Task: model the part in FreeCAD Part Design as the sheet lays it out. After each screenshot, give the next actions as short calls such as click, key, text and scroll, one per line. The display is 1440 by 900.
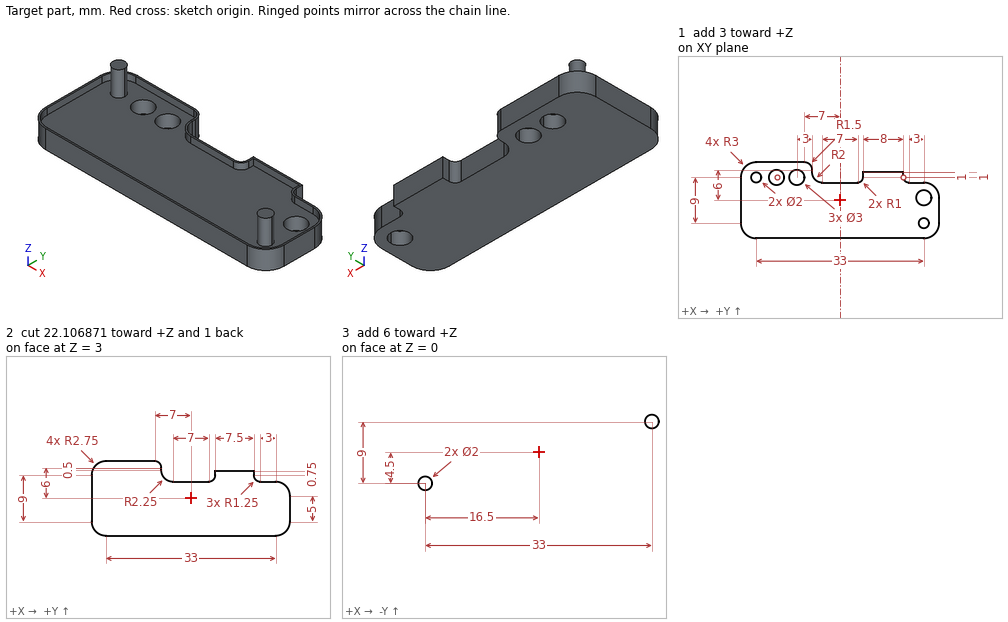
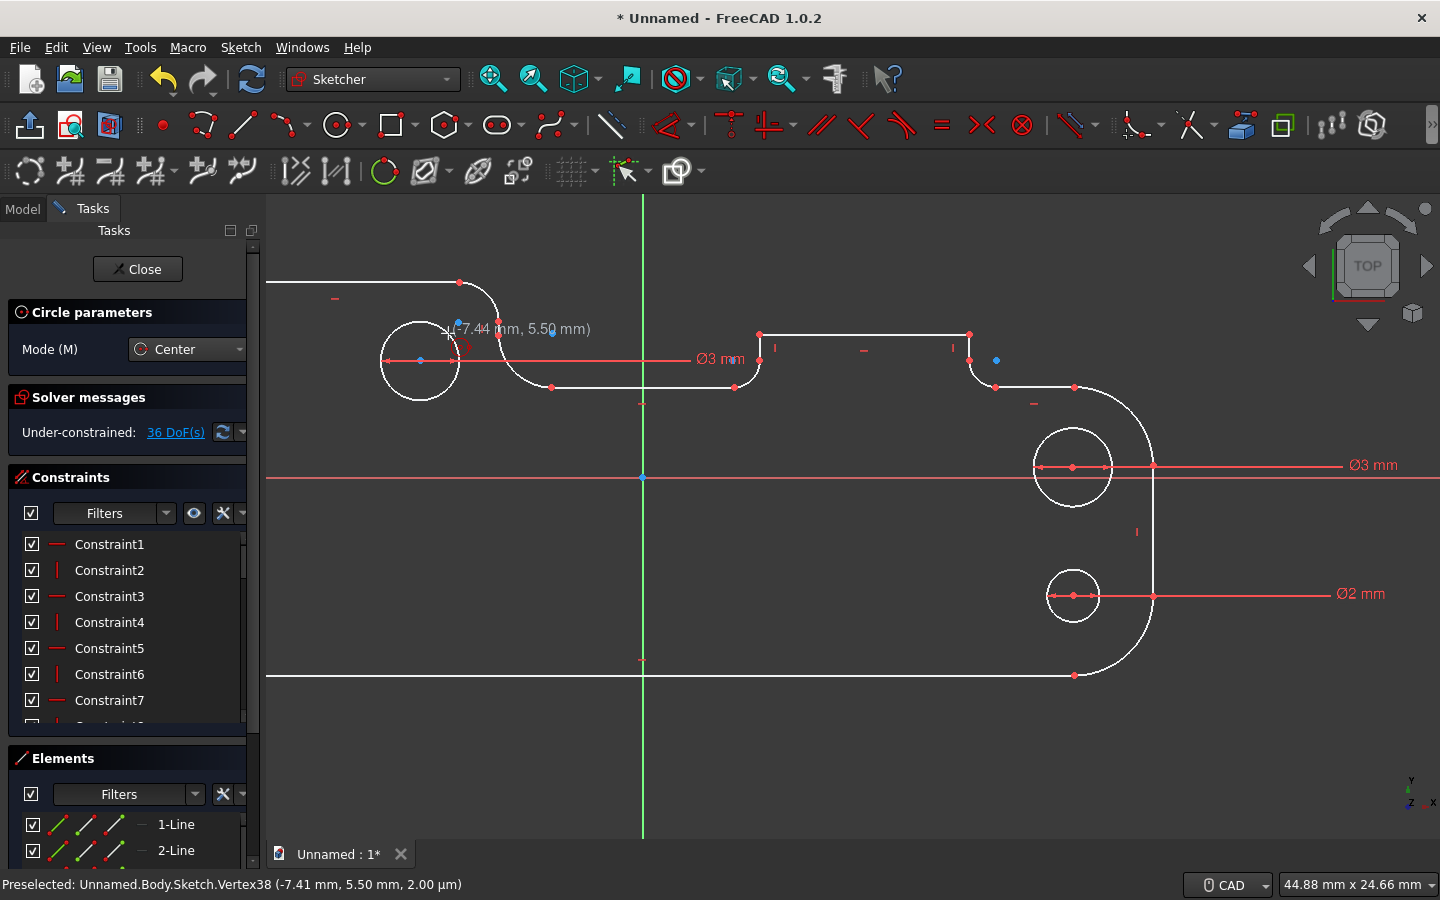
click(316, 360)
move(343, 333)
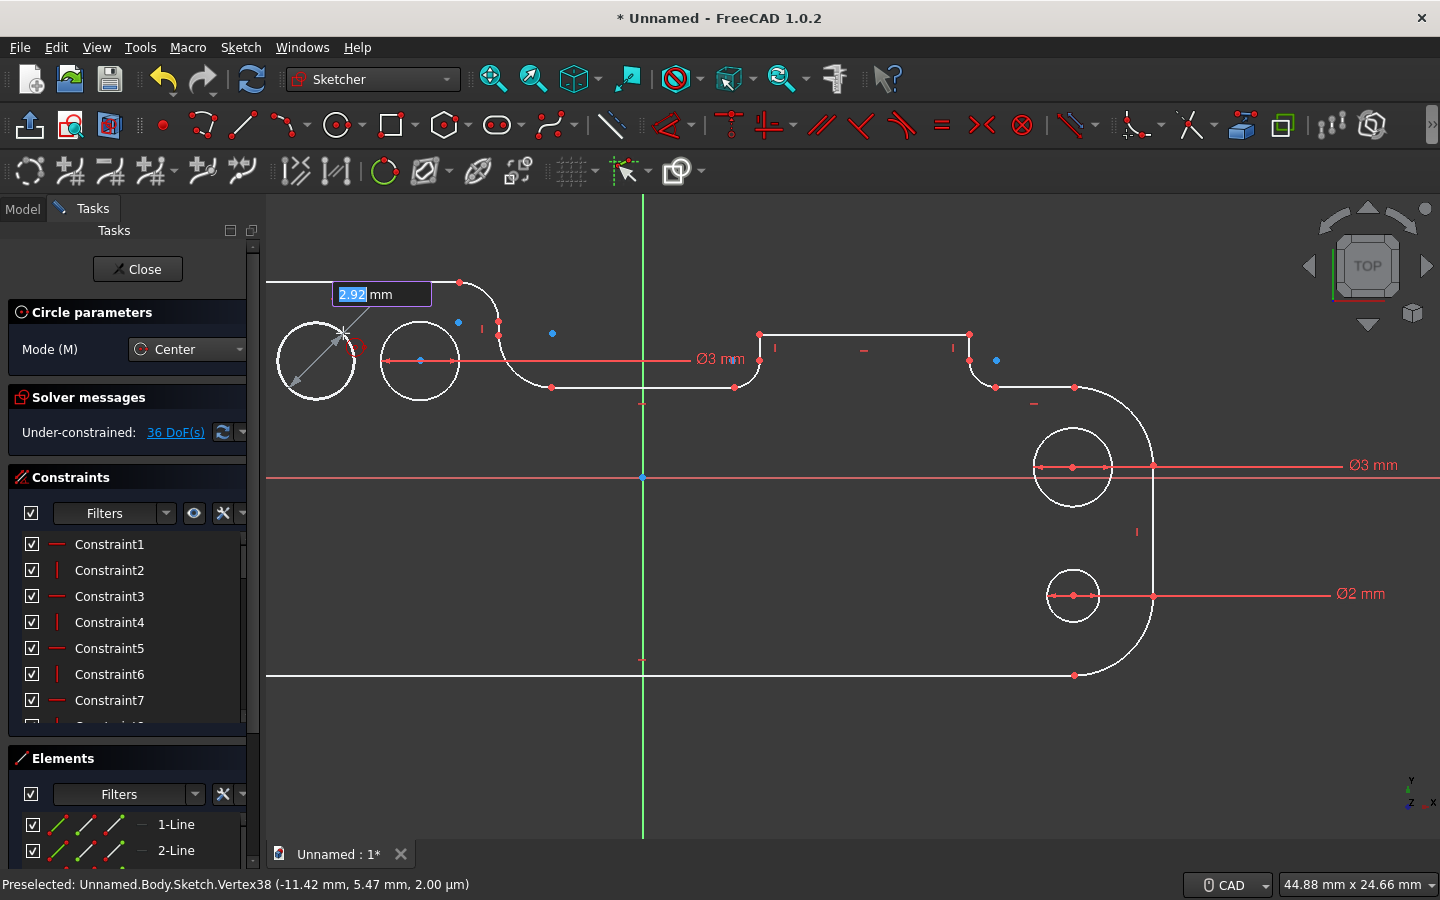
text(3)
key(Return)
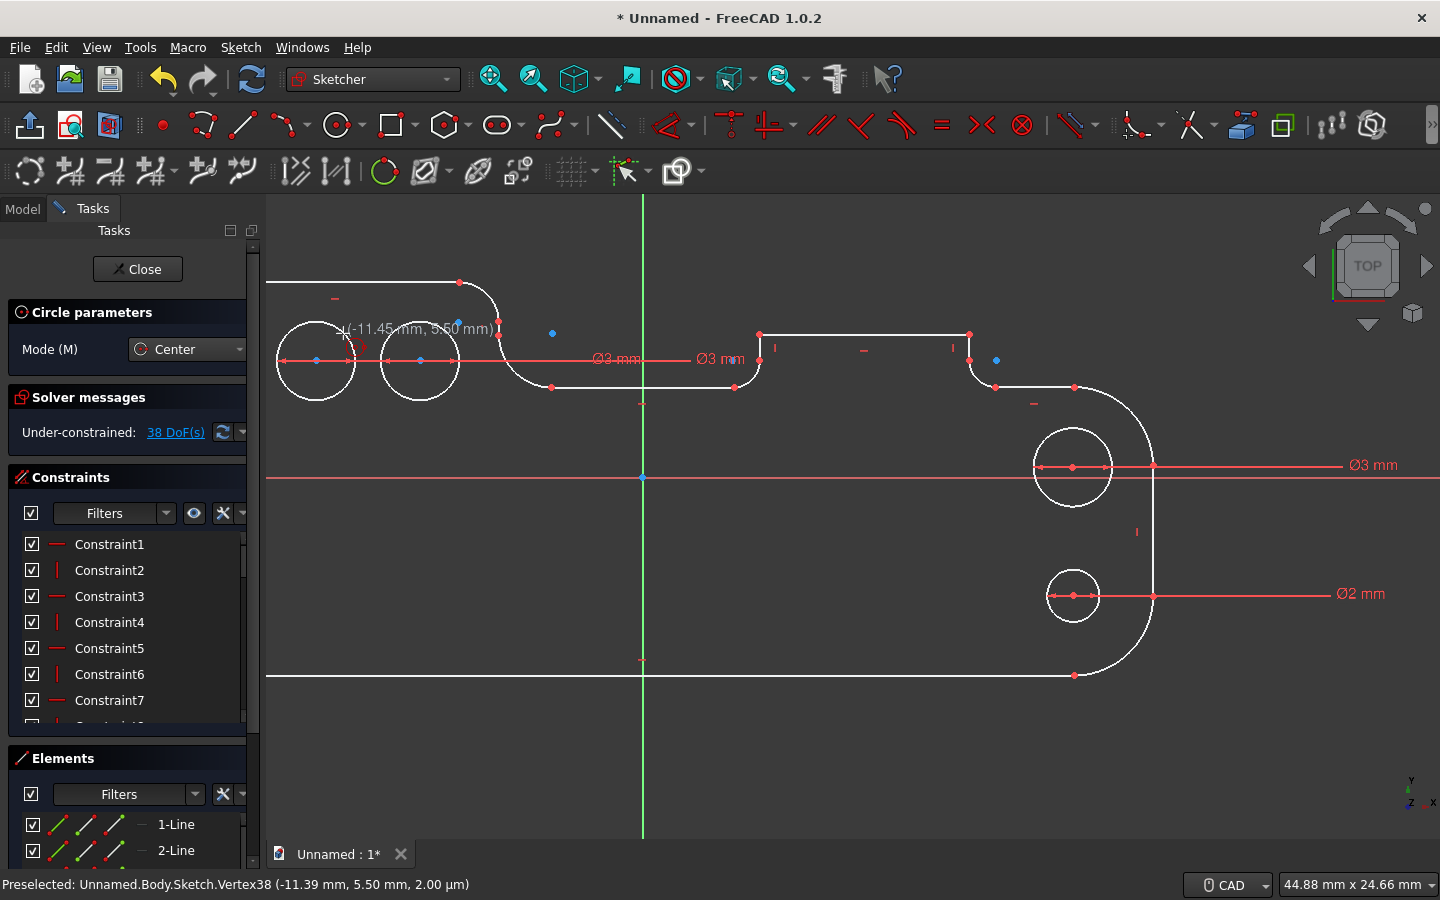
scroll(1073, 595, down, 2)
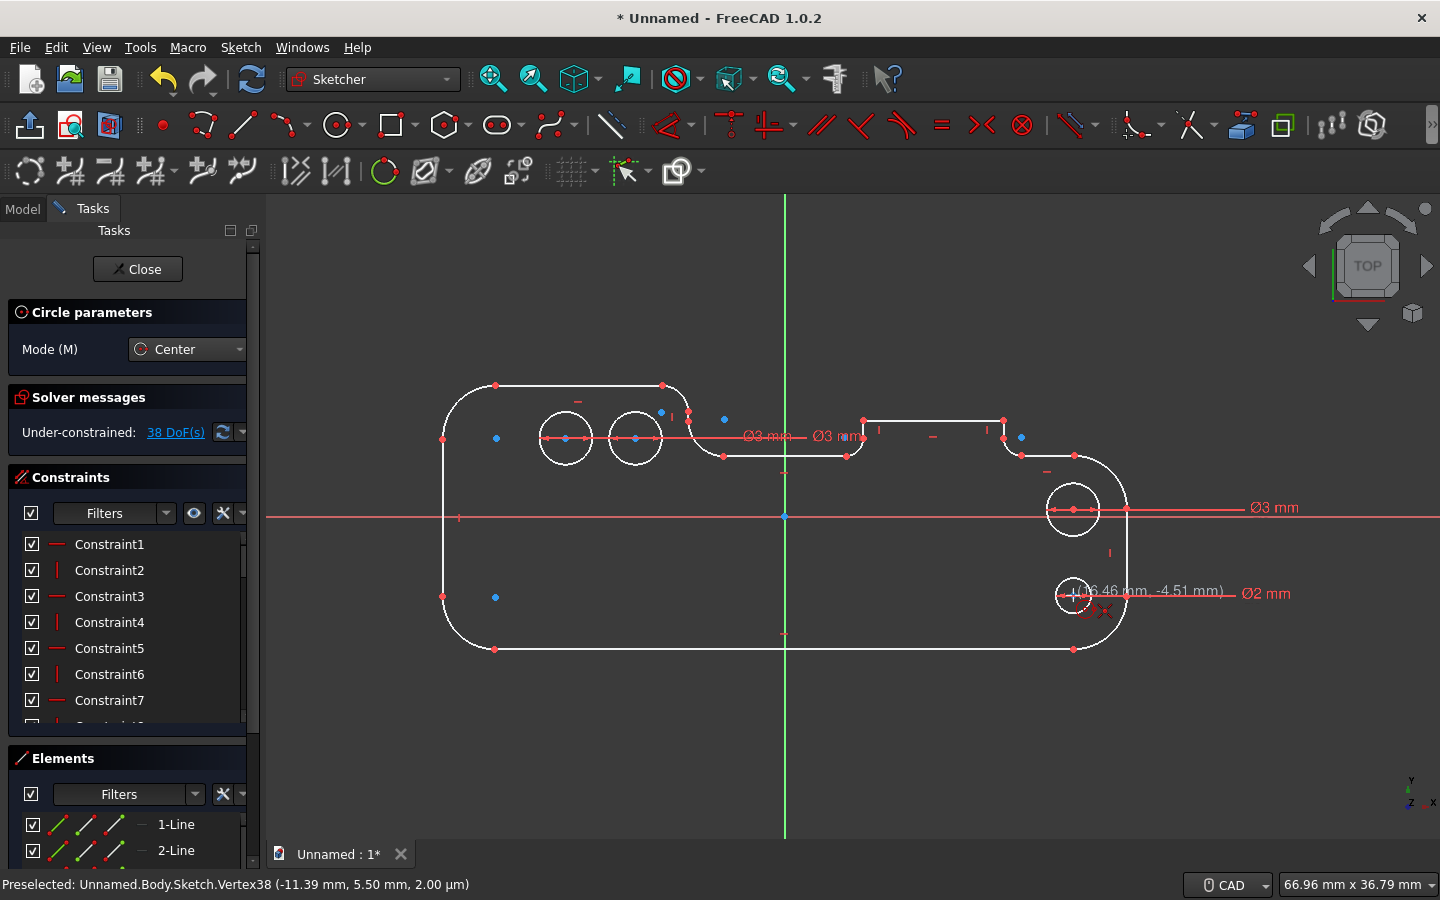
scroll(495, 438, up, 2)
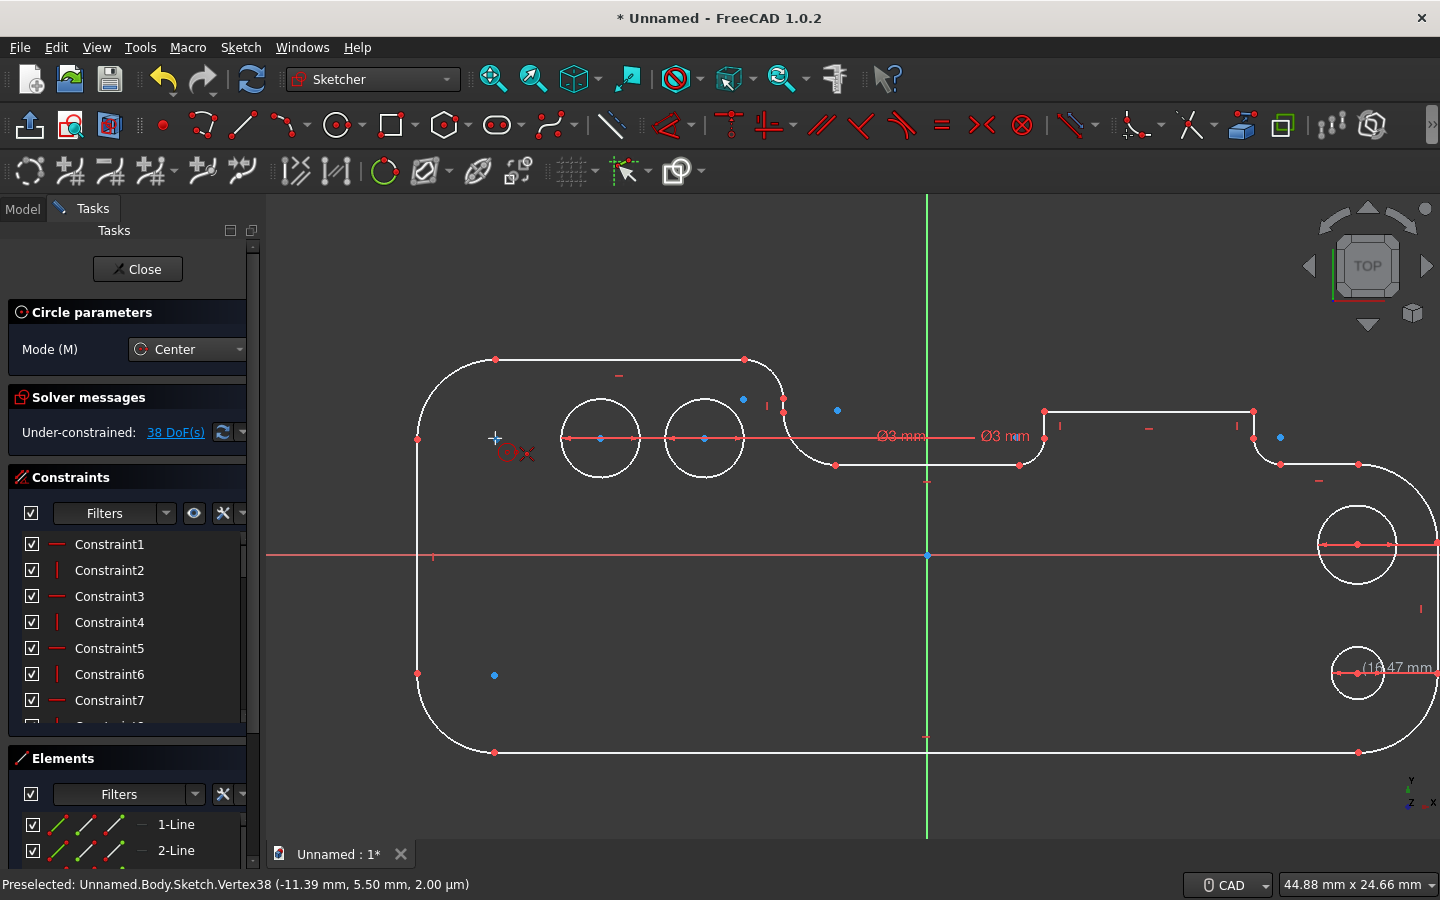
click(495, 438)
move(514, 419)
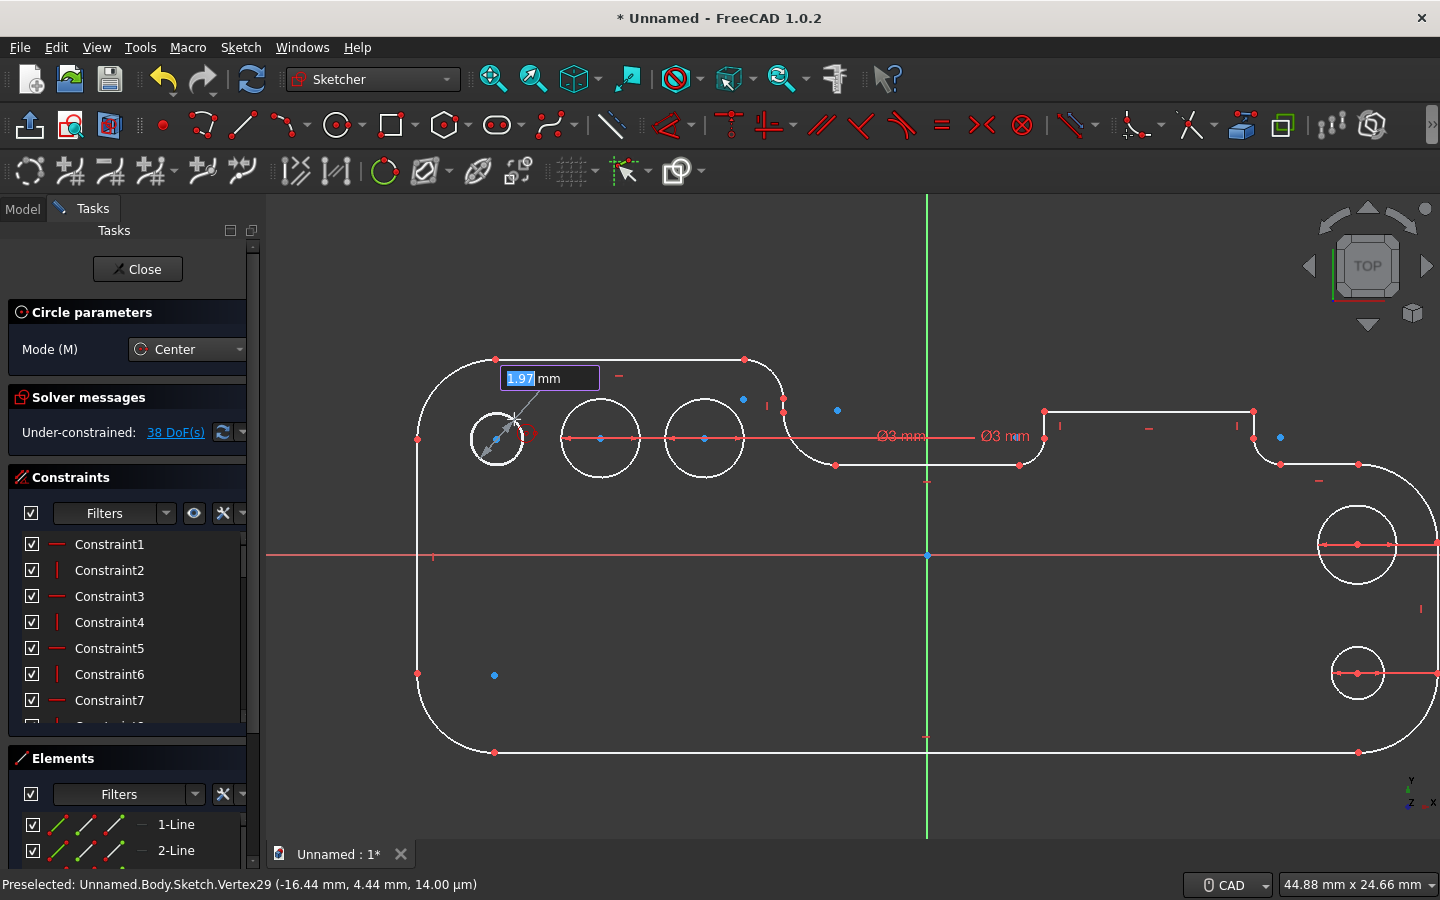
text(2)
key(Return)
key(Escape)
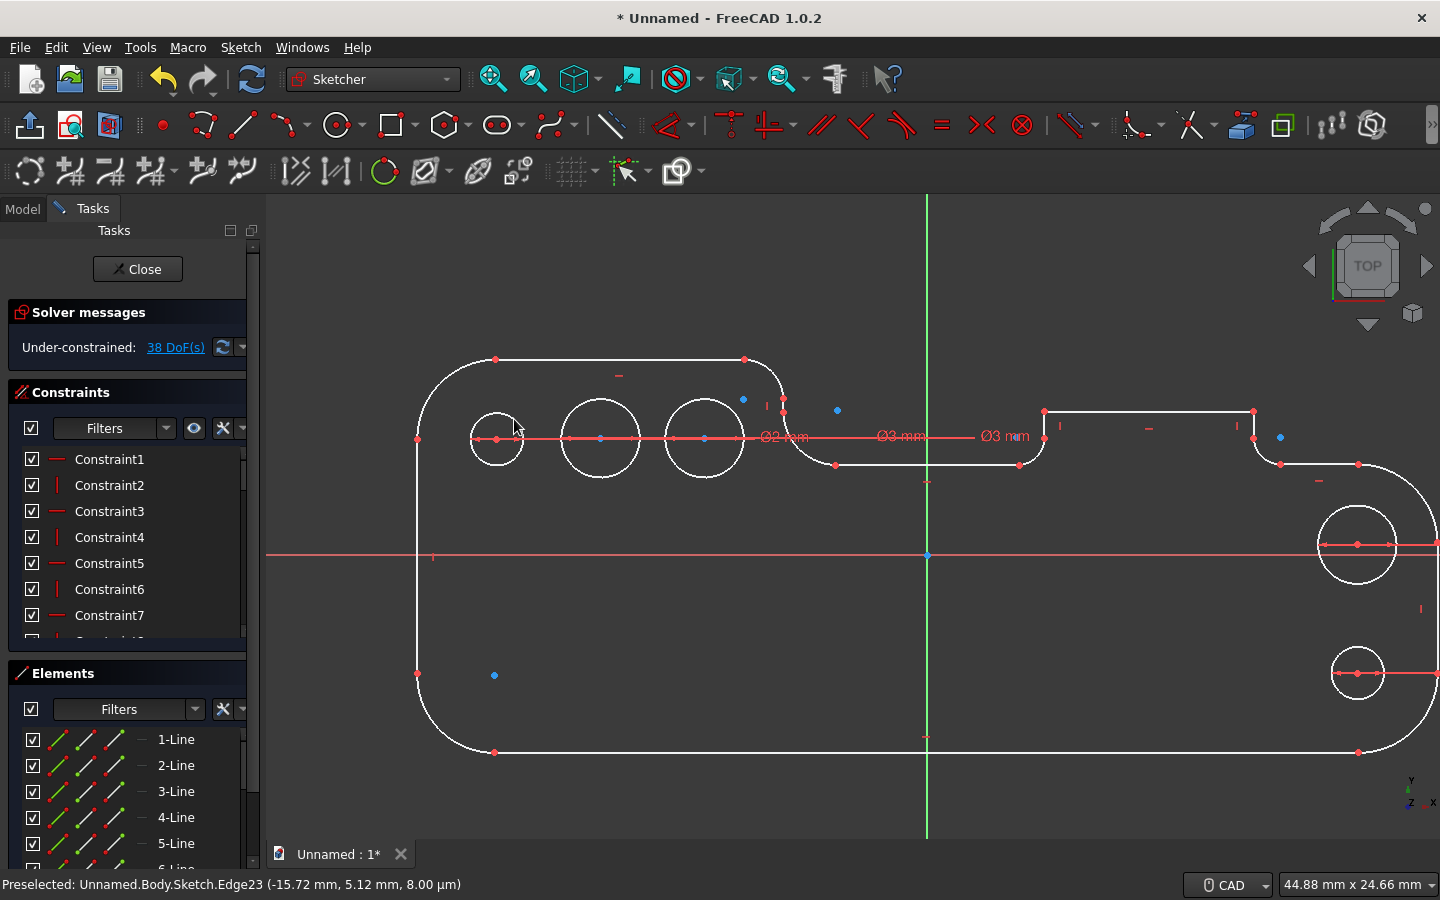
click(964, 465)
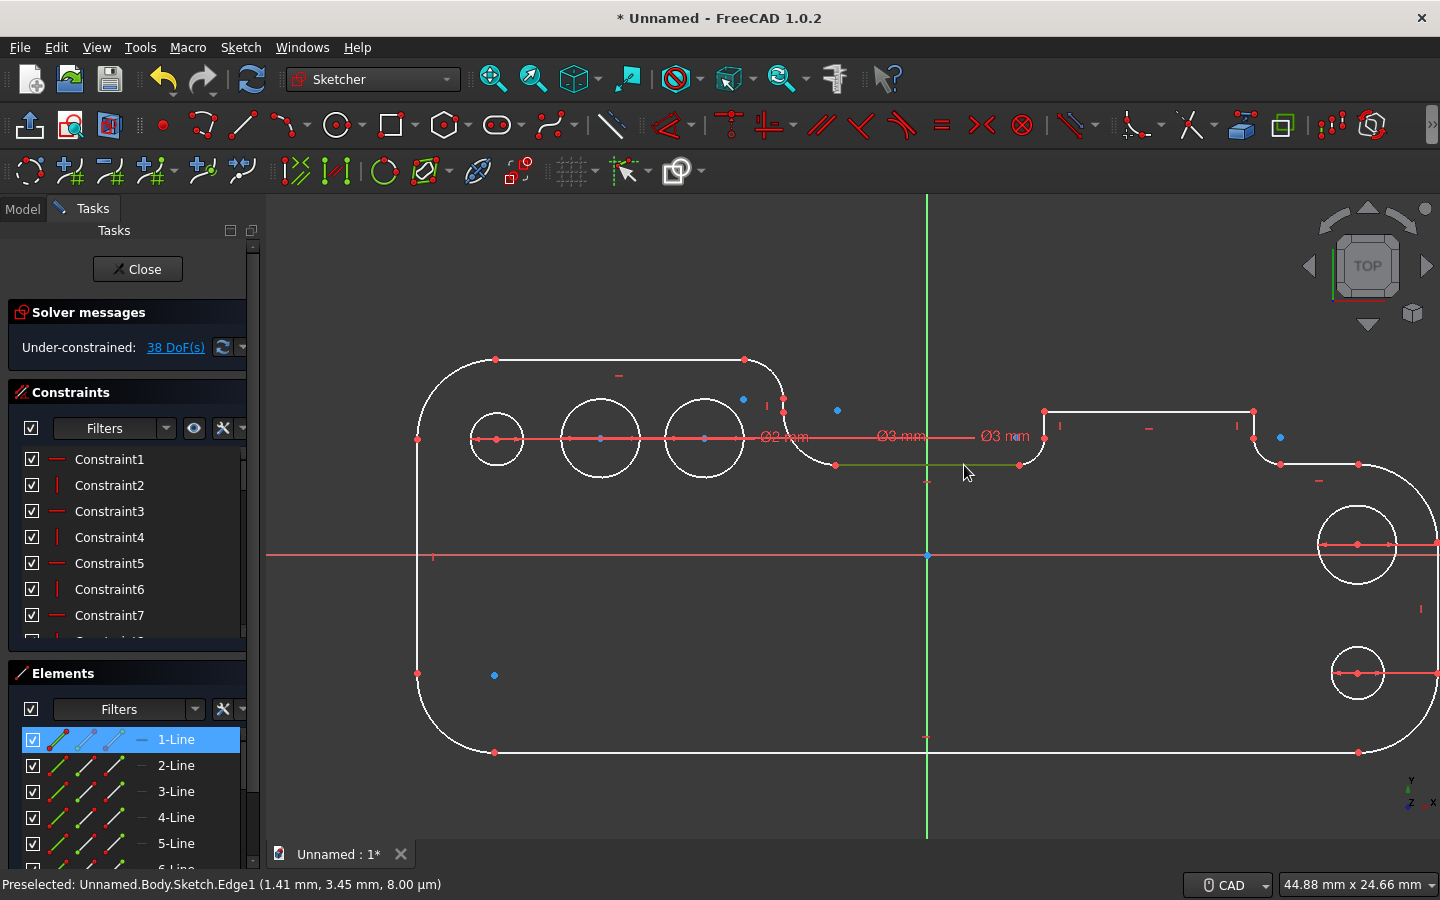
click(812, 459)